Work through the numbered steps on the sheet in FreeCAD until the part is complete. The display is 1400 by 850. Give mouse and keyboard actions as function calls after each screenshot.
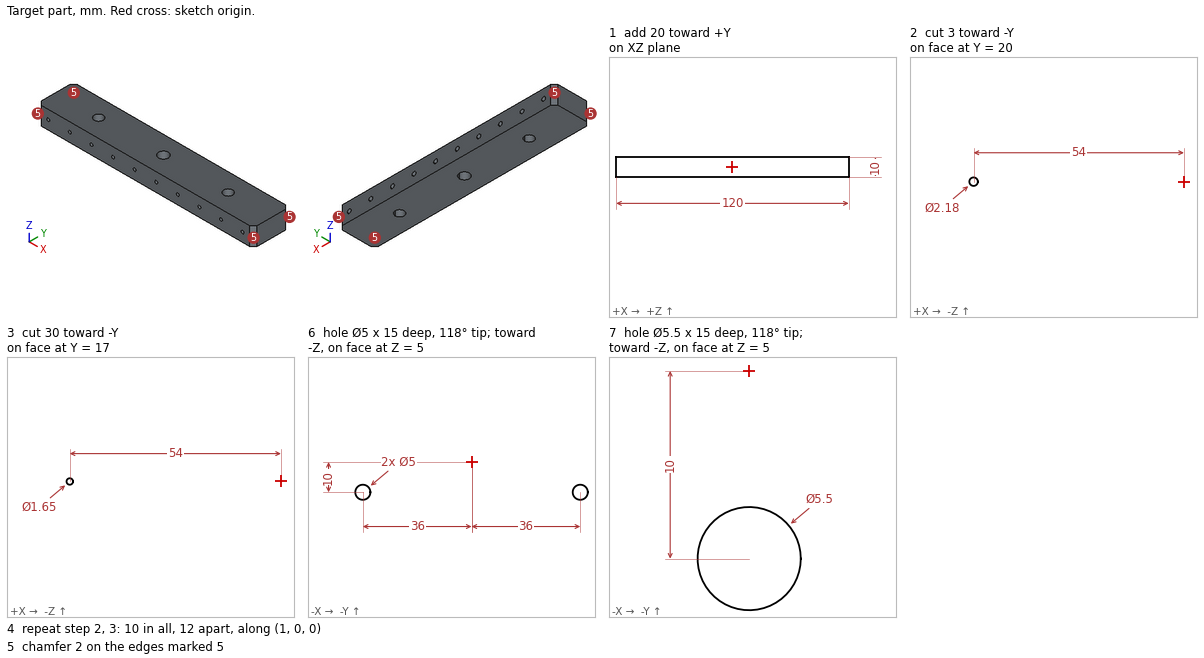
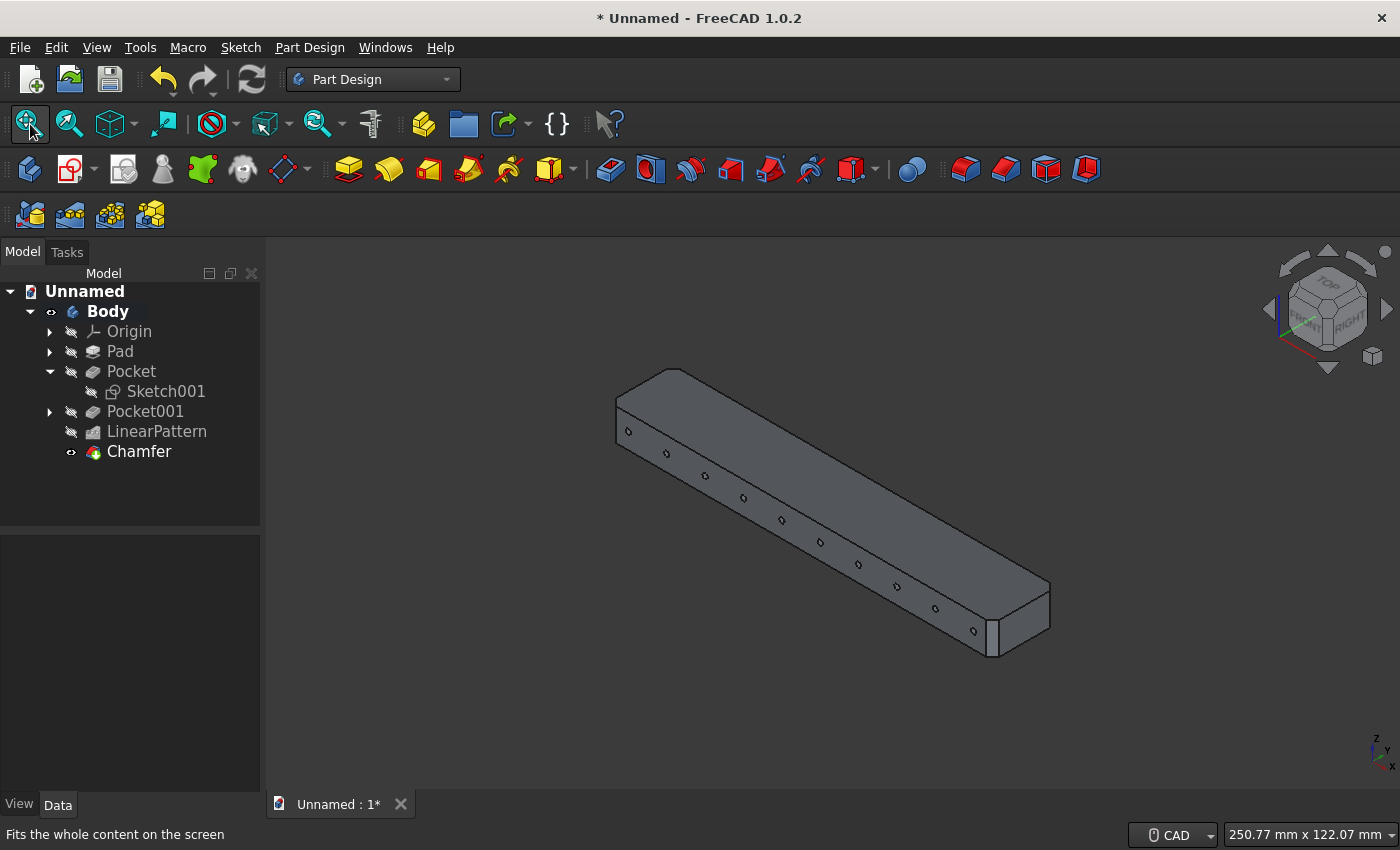
click(943, 557)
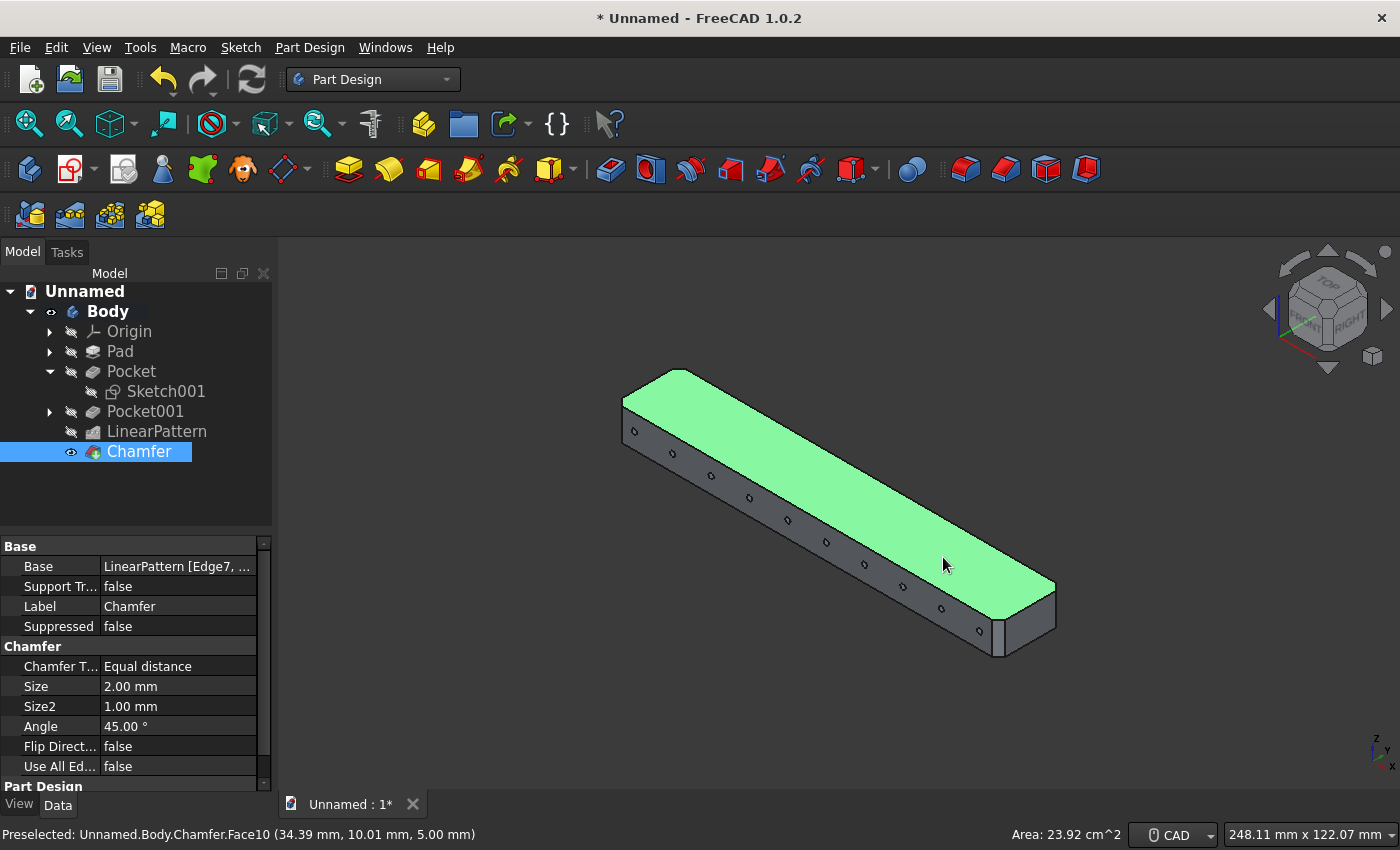
click(70, 170)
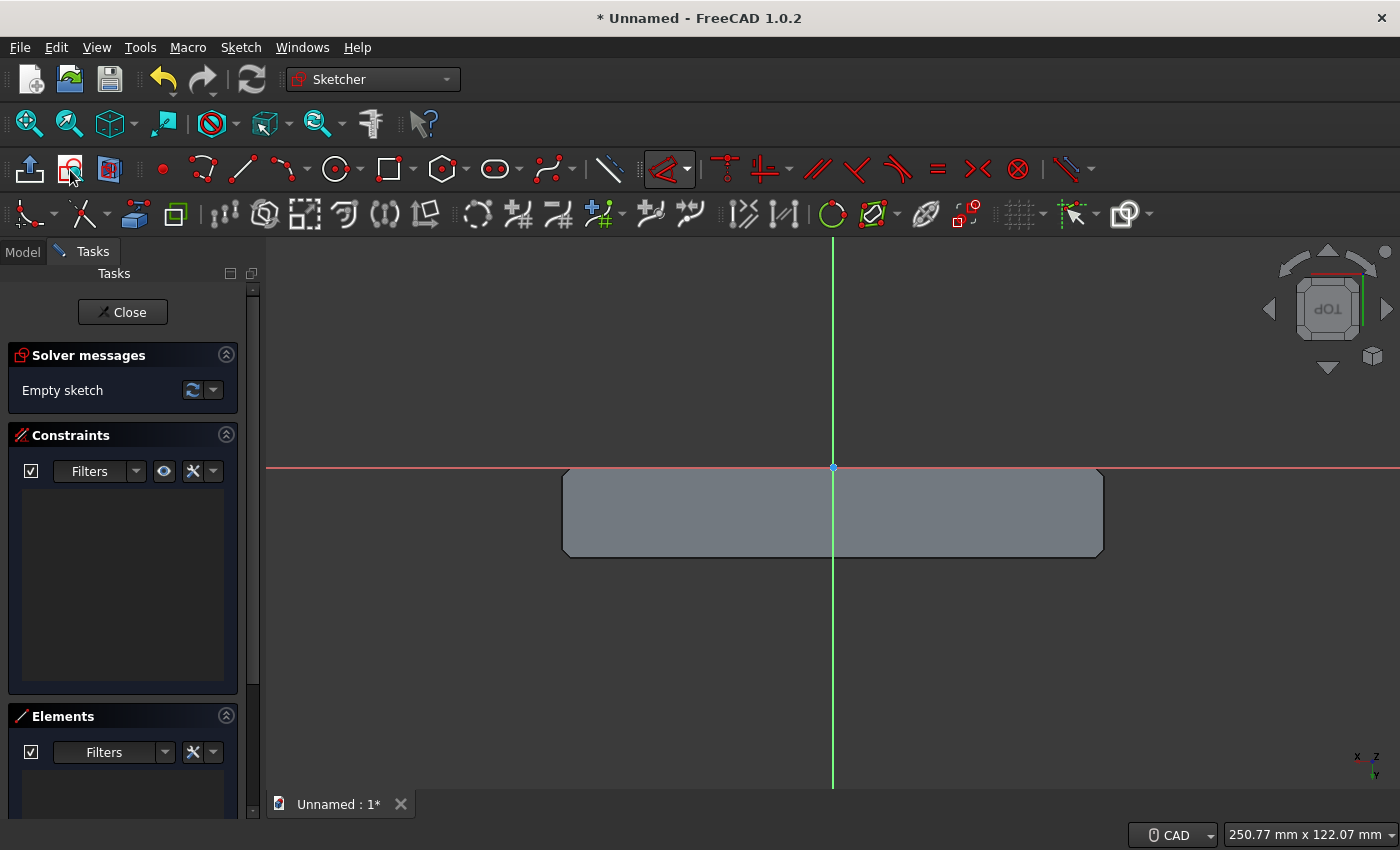
scroll(916, 475, up, 3)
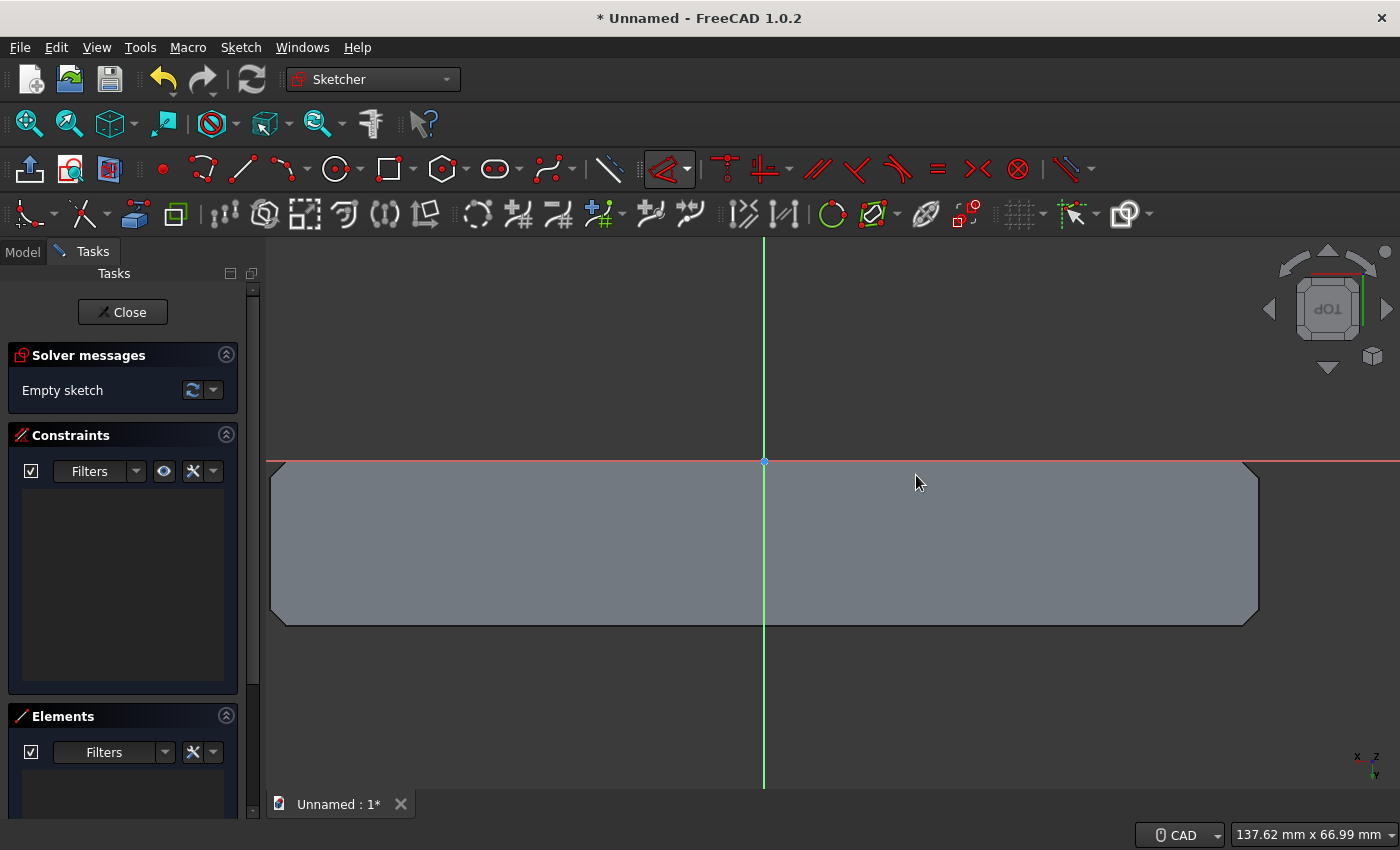
click(336, 170)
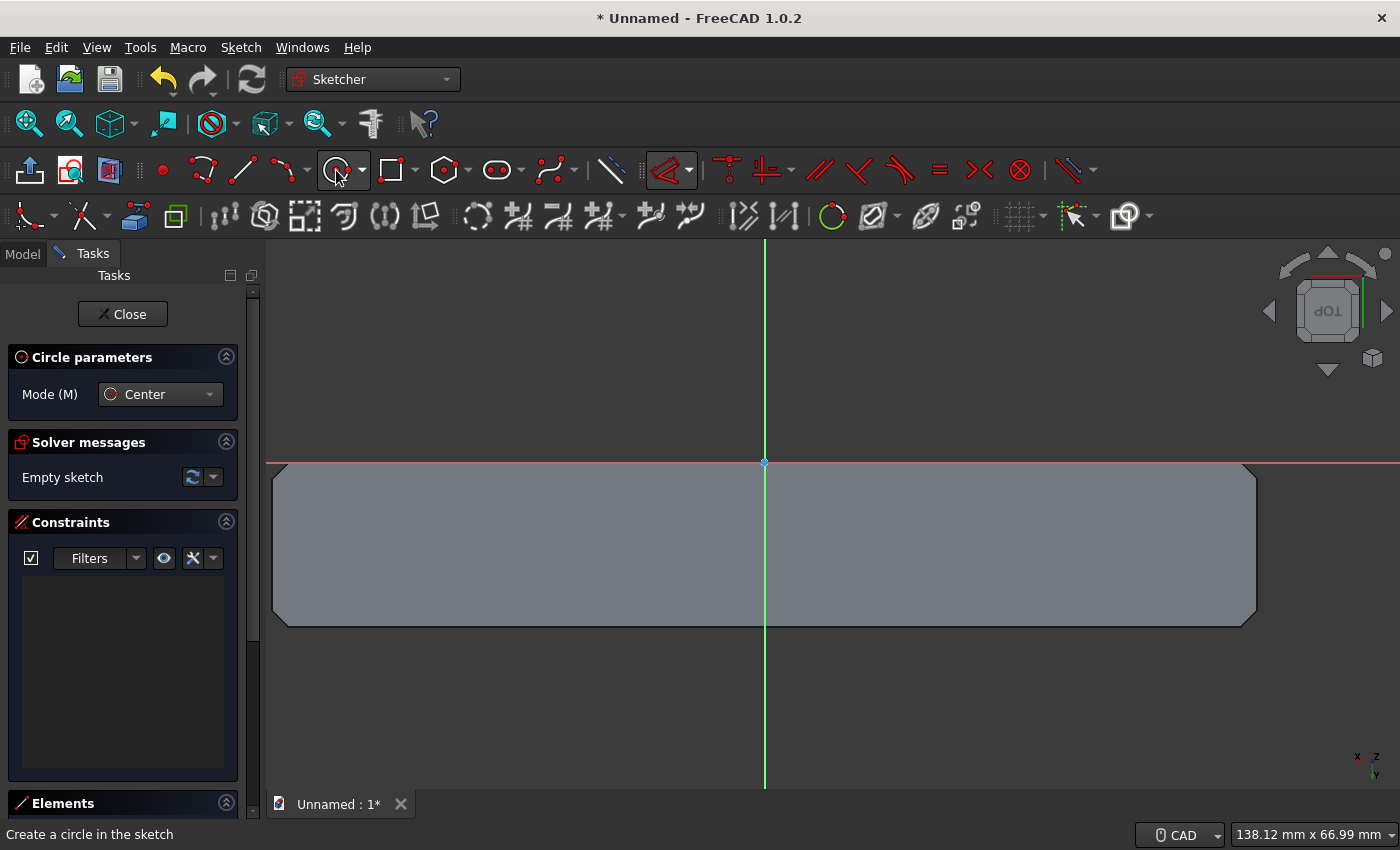
click(469, 545)
click(483, 530)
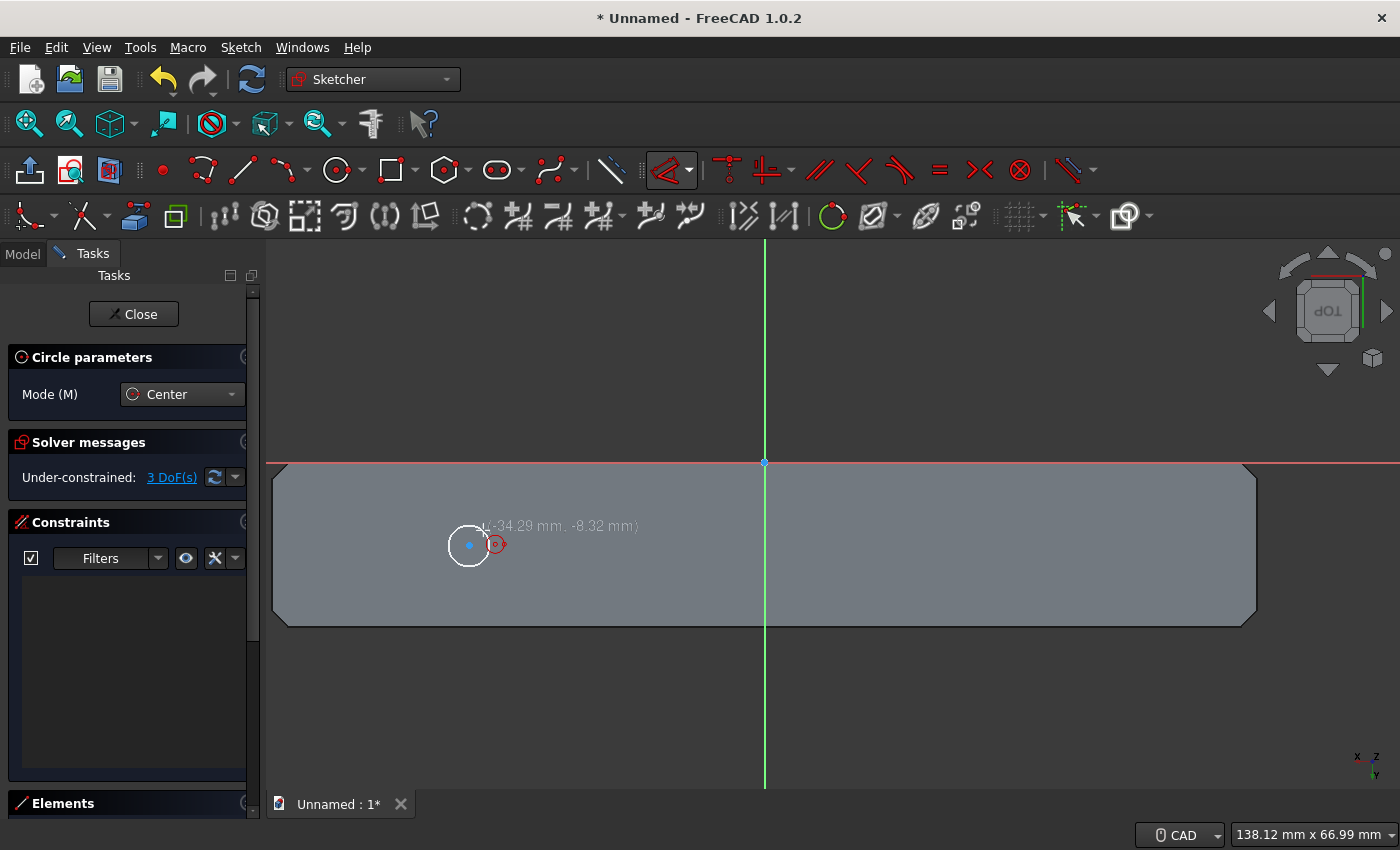
click(1060, 545)
click(1075, 530)
key(Escape)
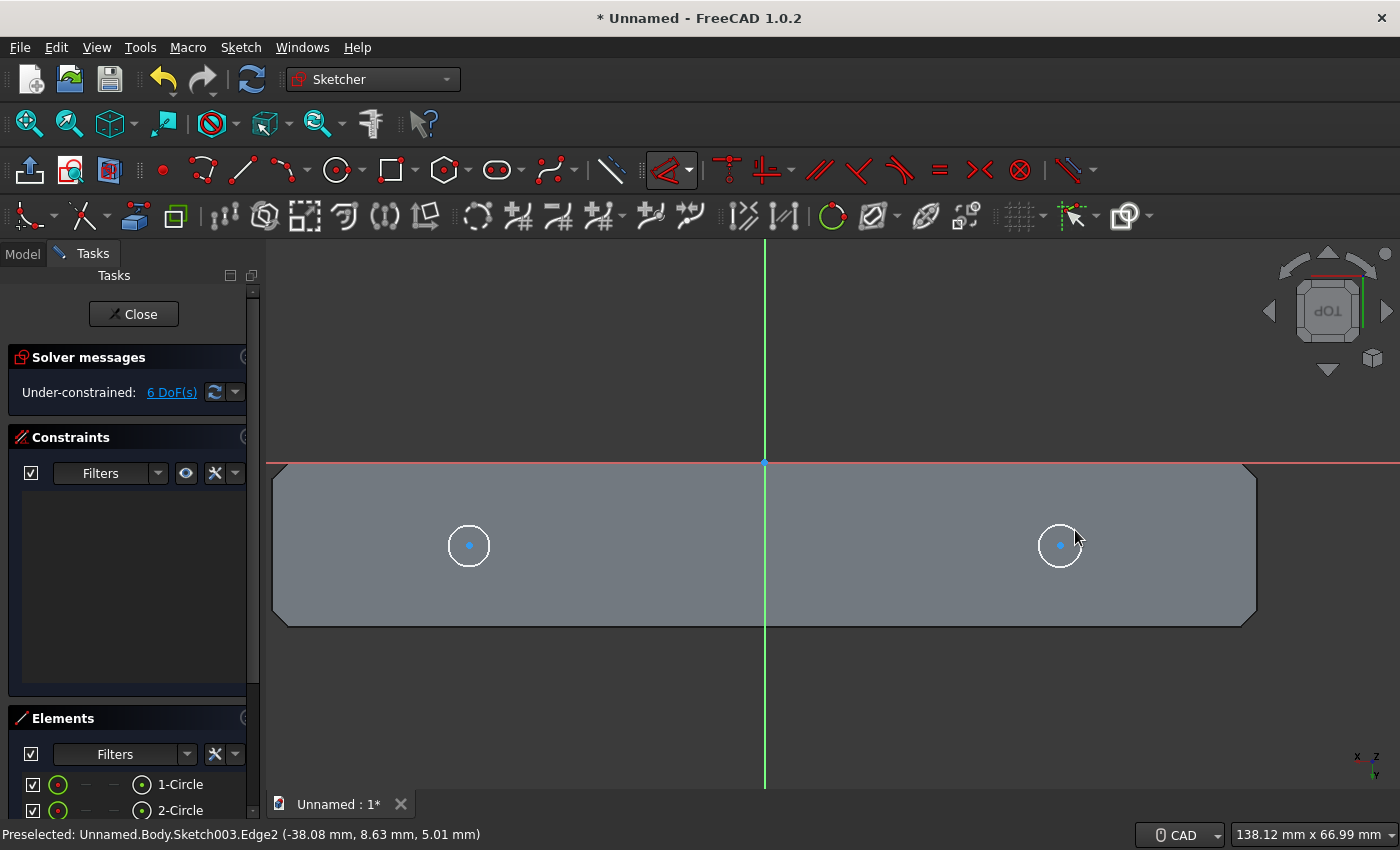
click(483, 531)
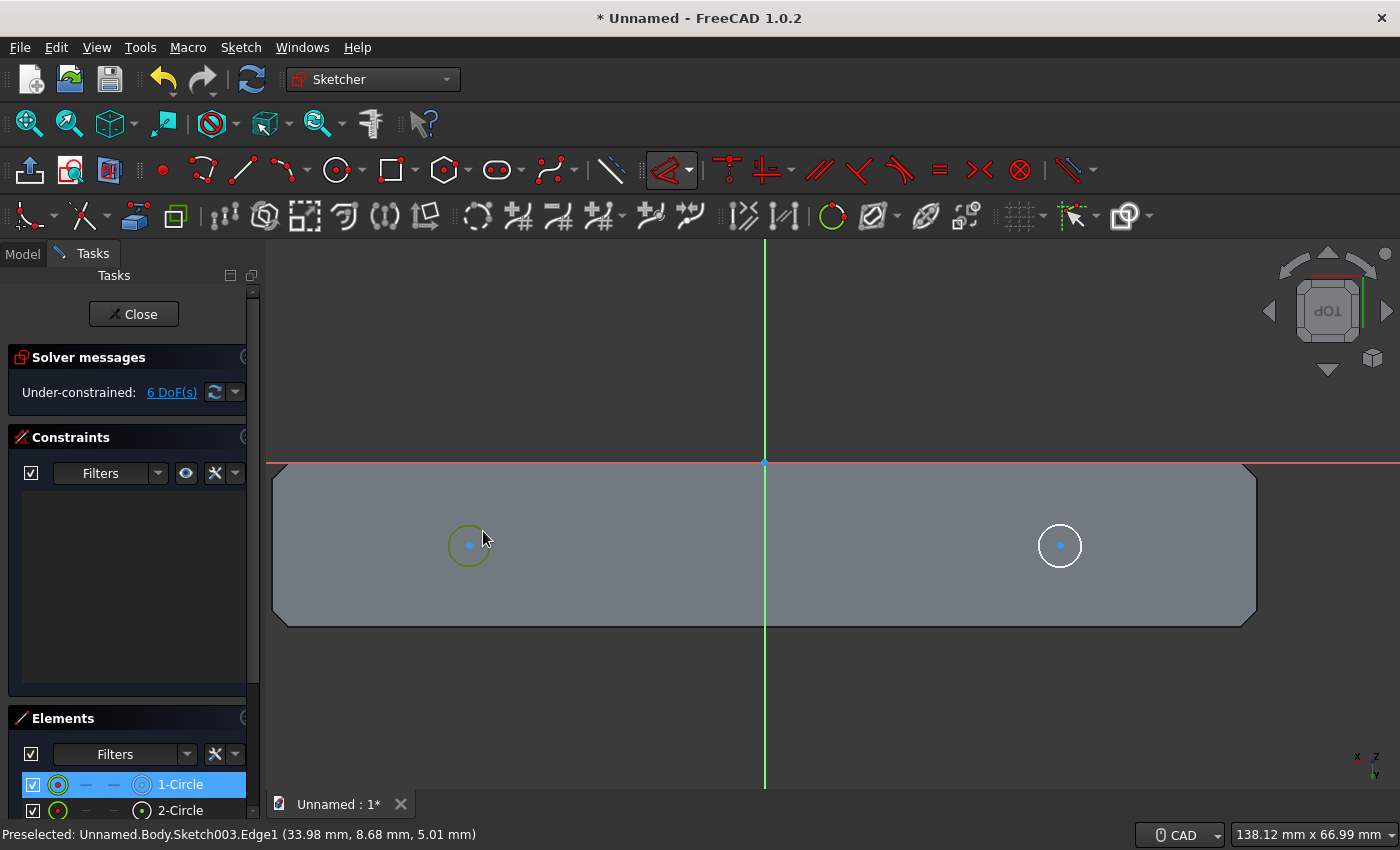
click(1075, 531)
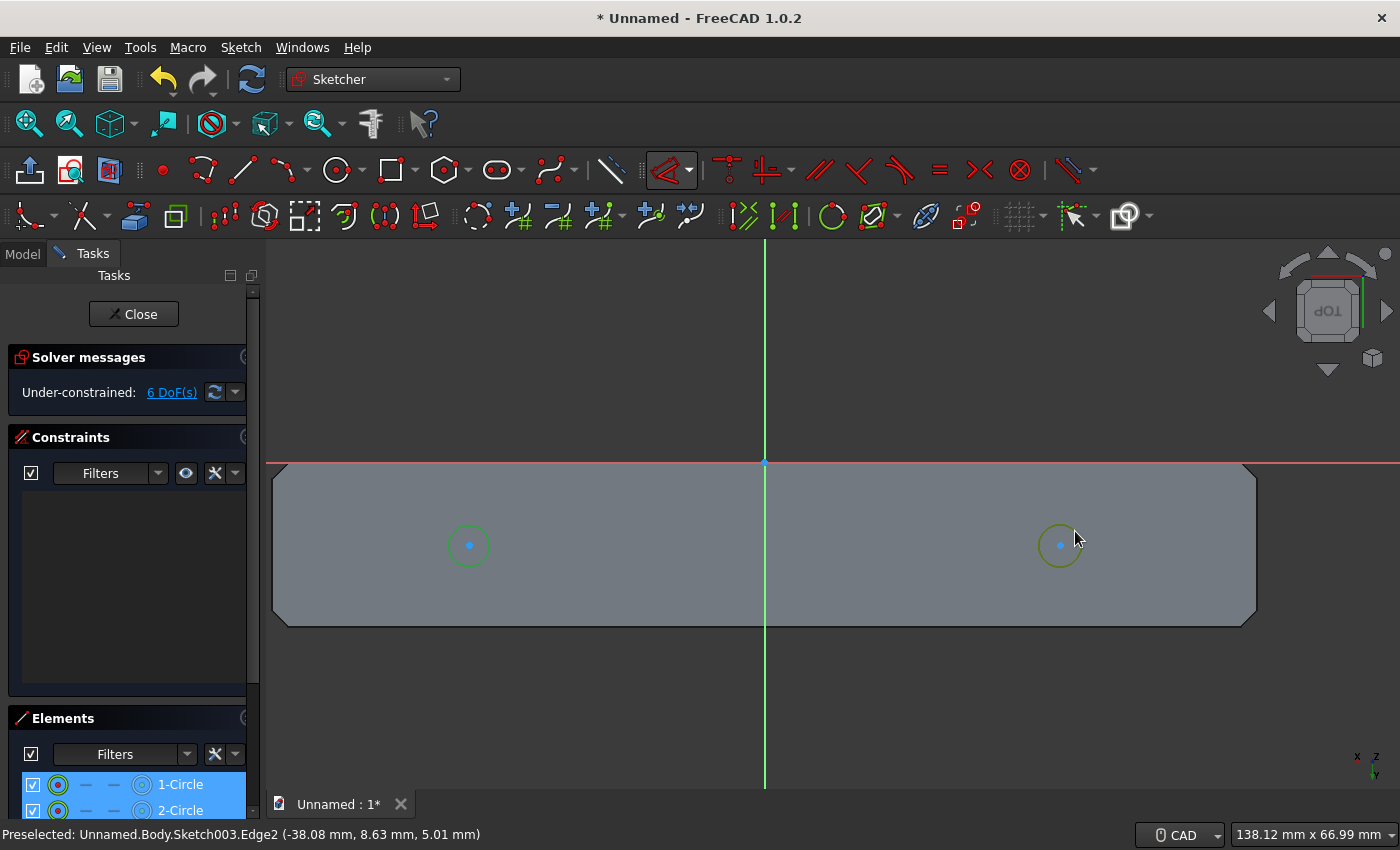
key(e)